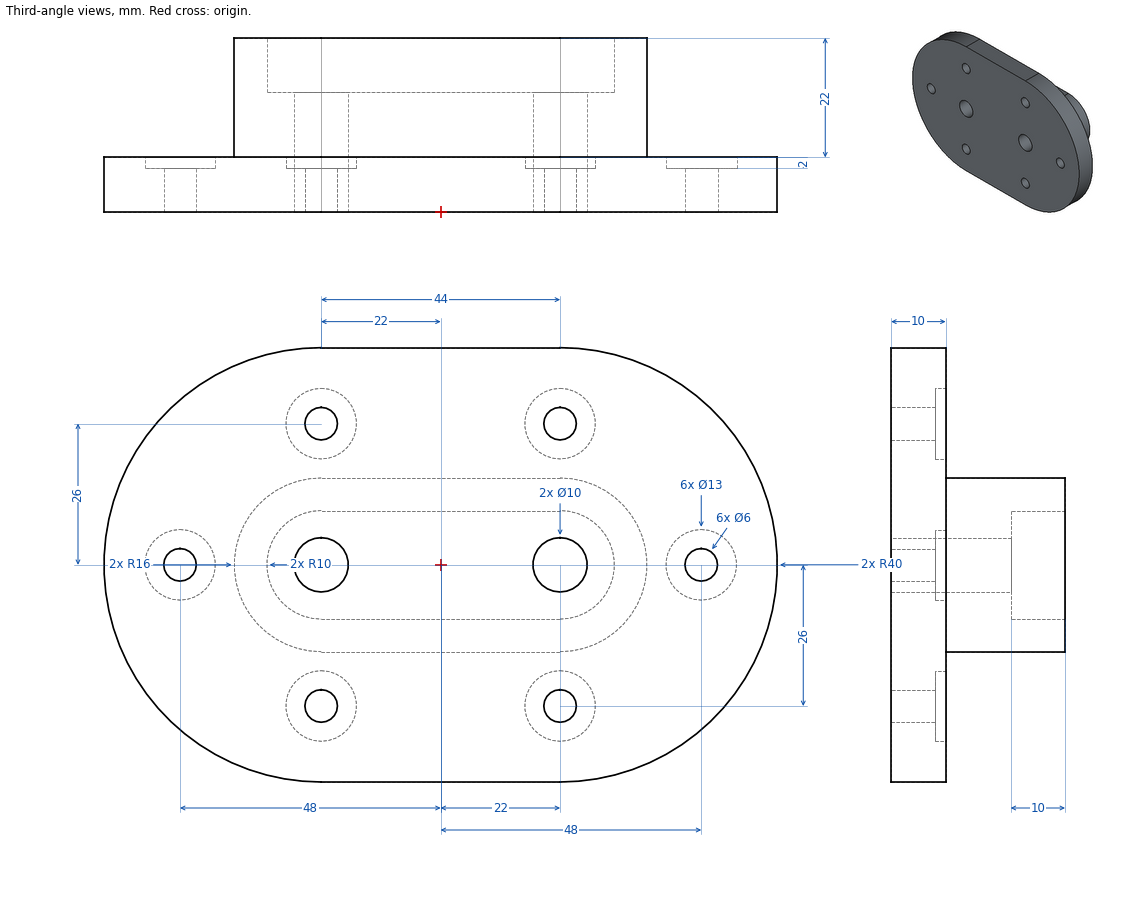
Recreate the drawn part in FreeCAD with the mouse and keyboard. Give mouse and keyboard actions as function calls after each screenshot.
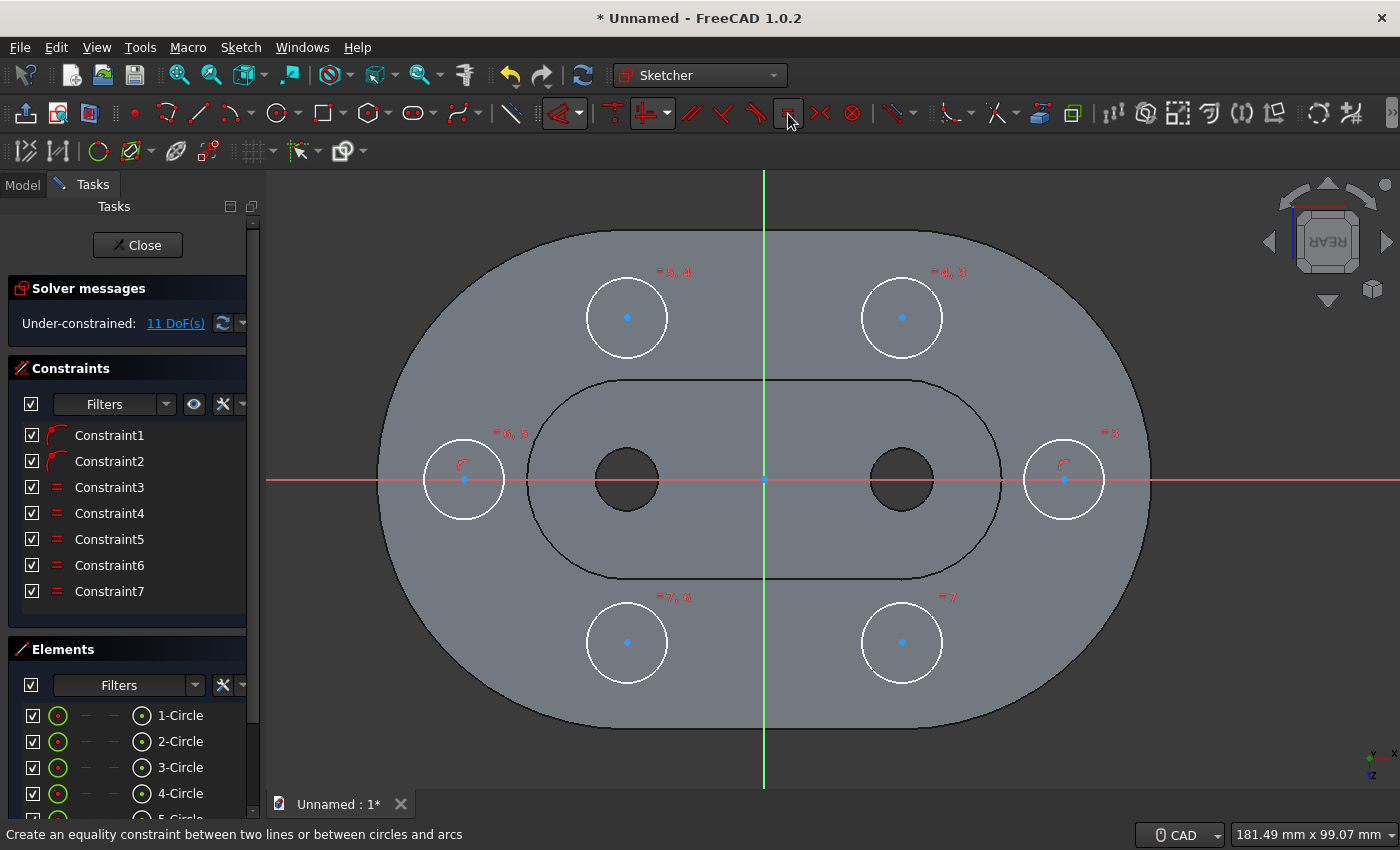
click(902, 318)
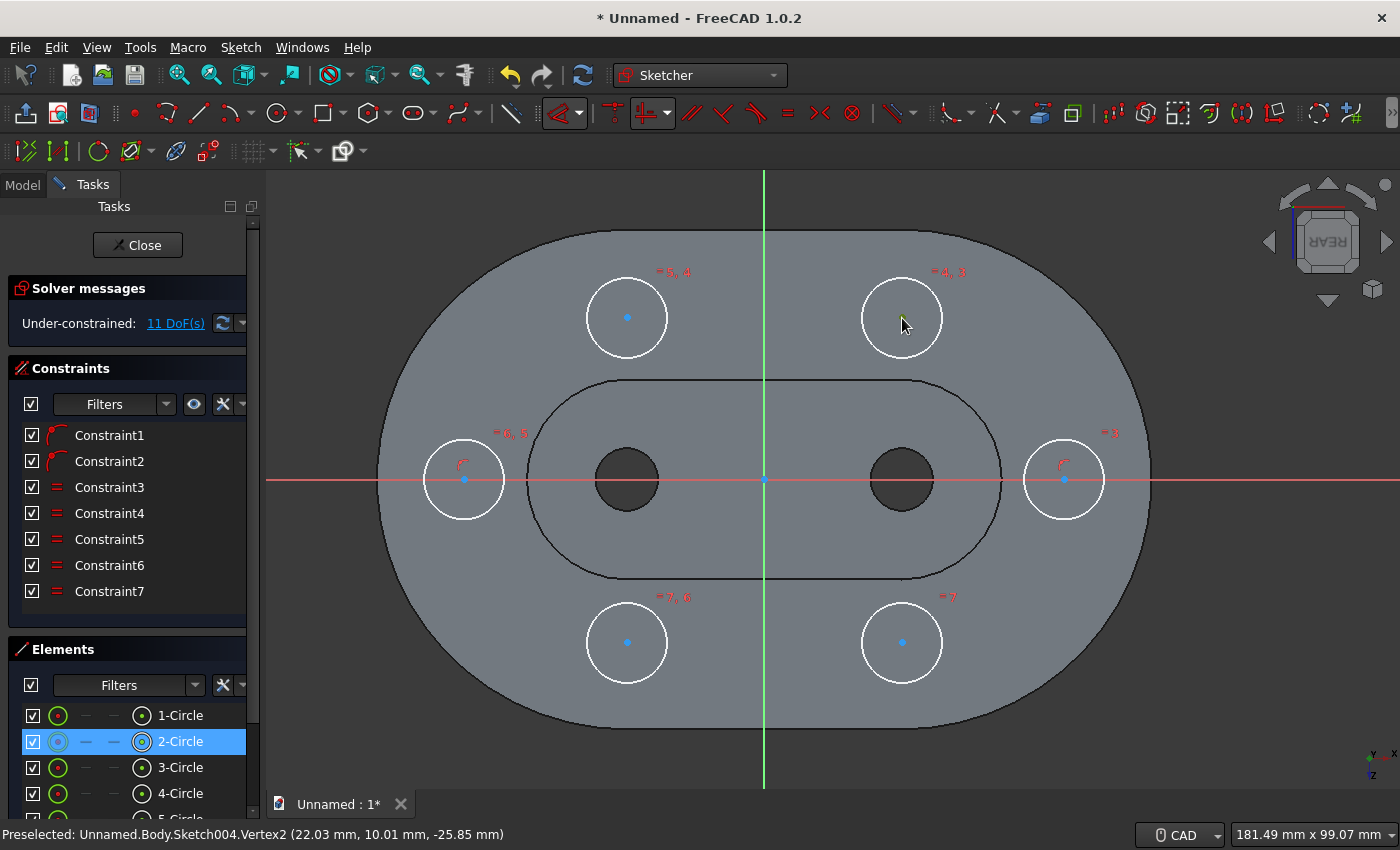
click(627, 318)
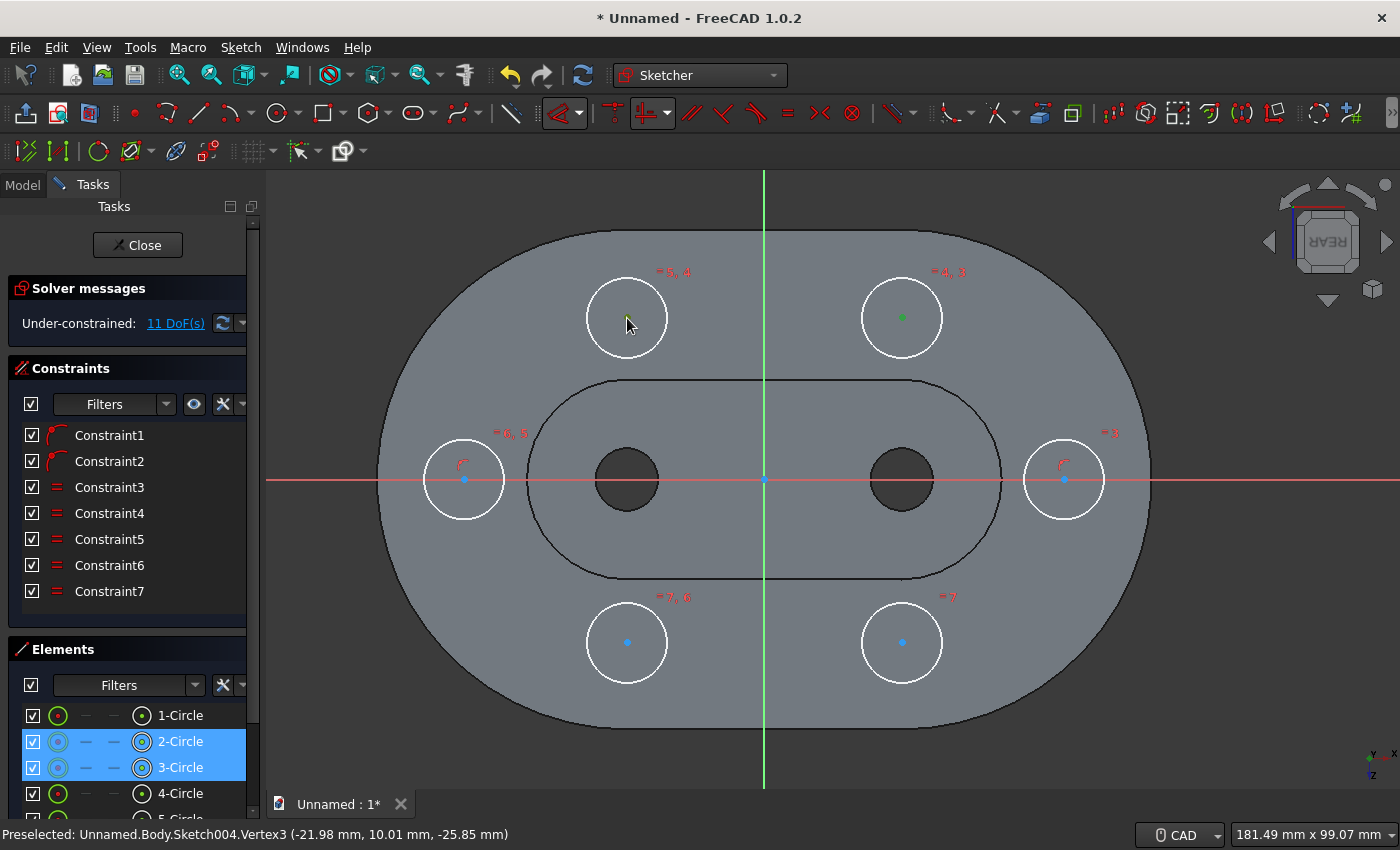
key(h)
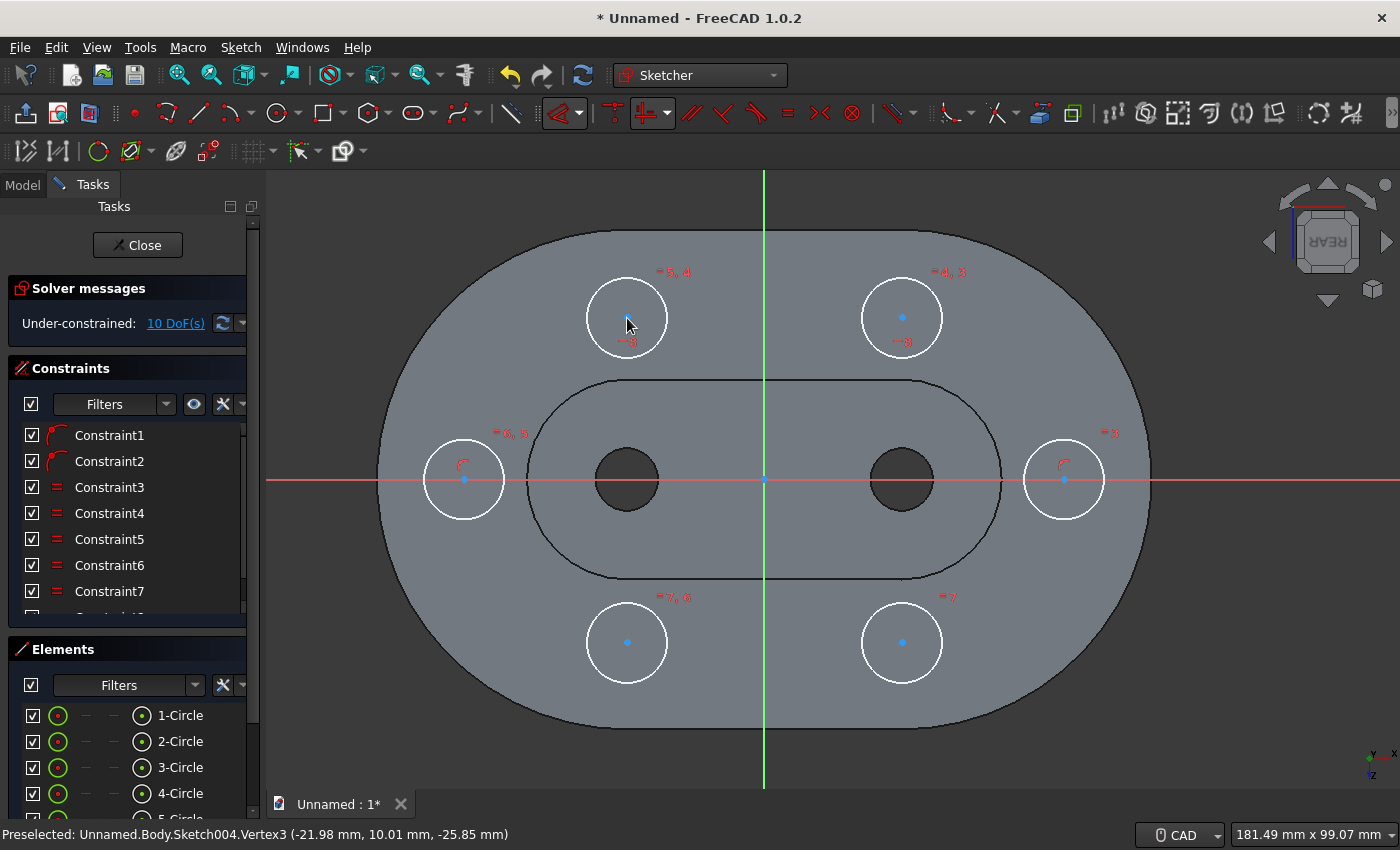
click(627, 318)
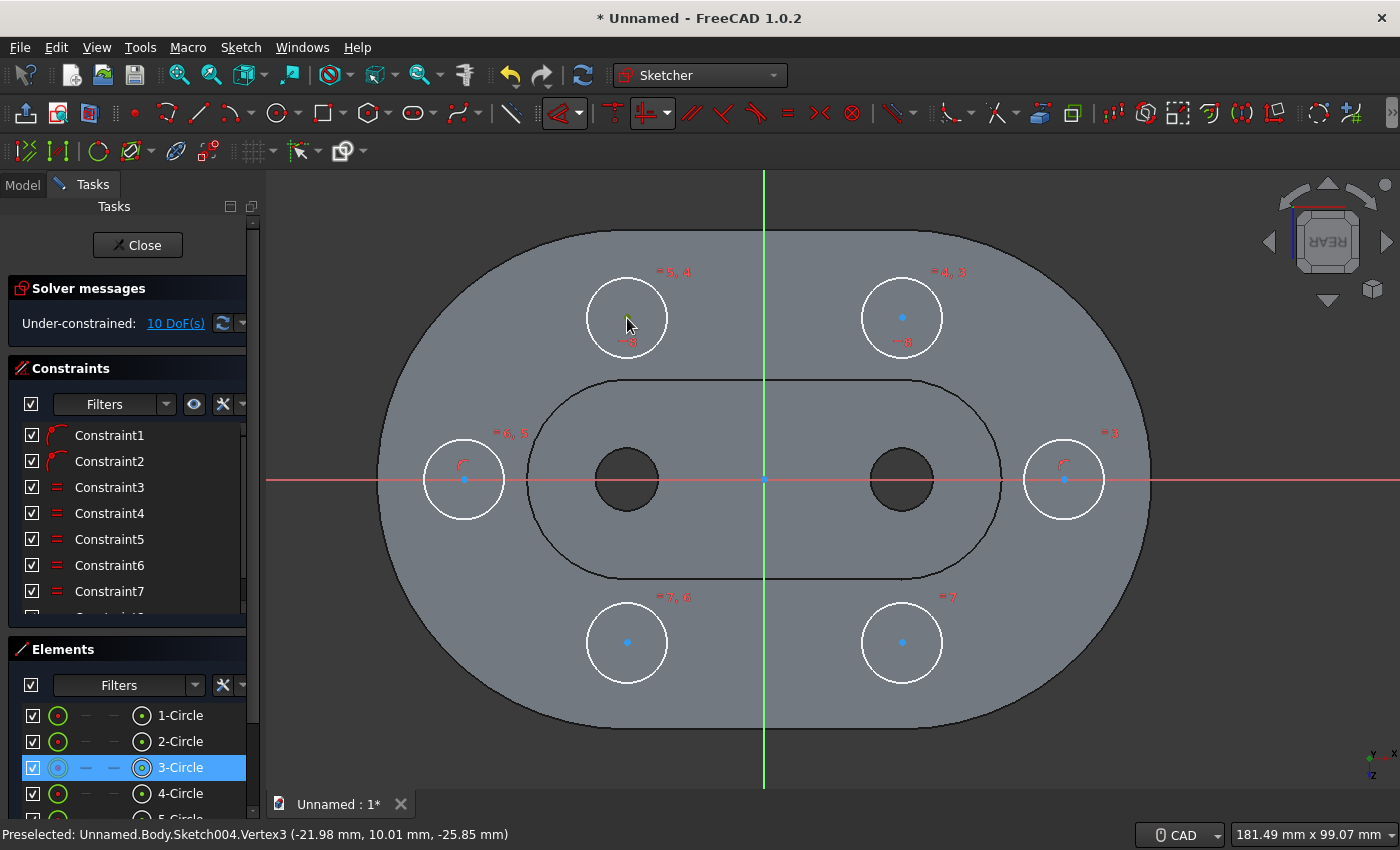
click(627, 643)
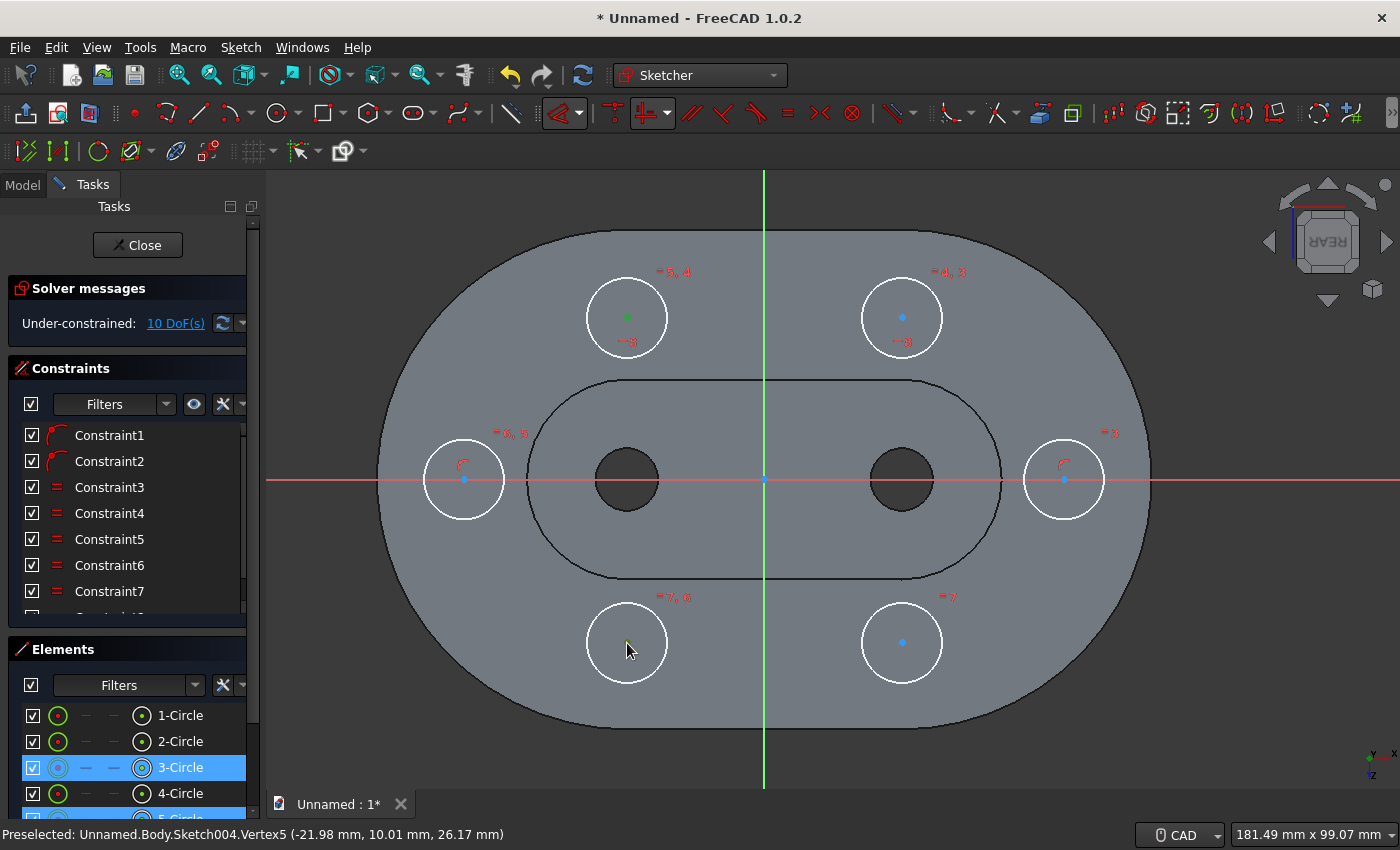
key(v)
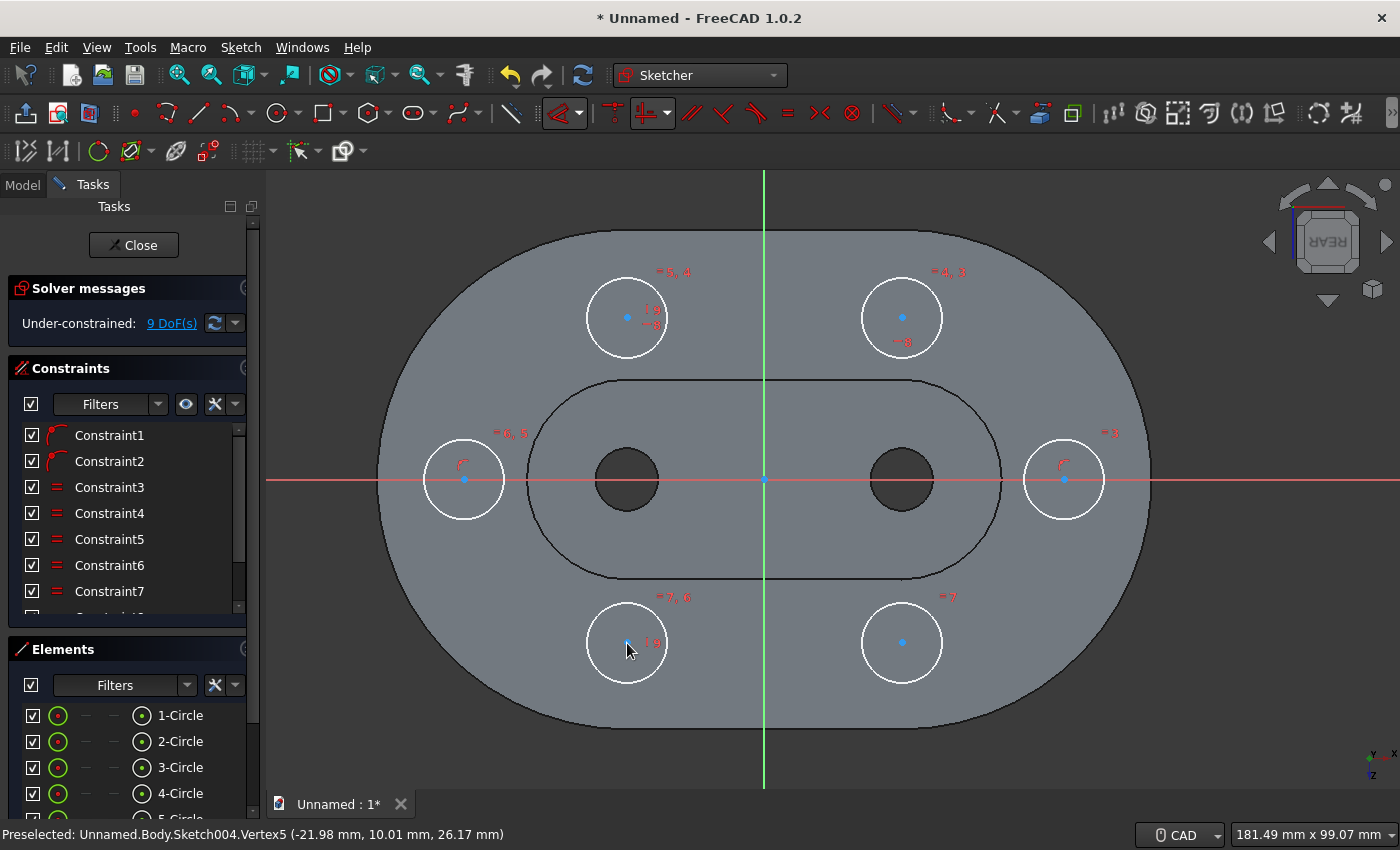
click(902, 318)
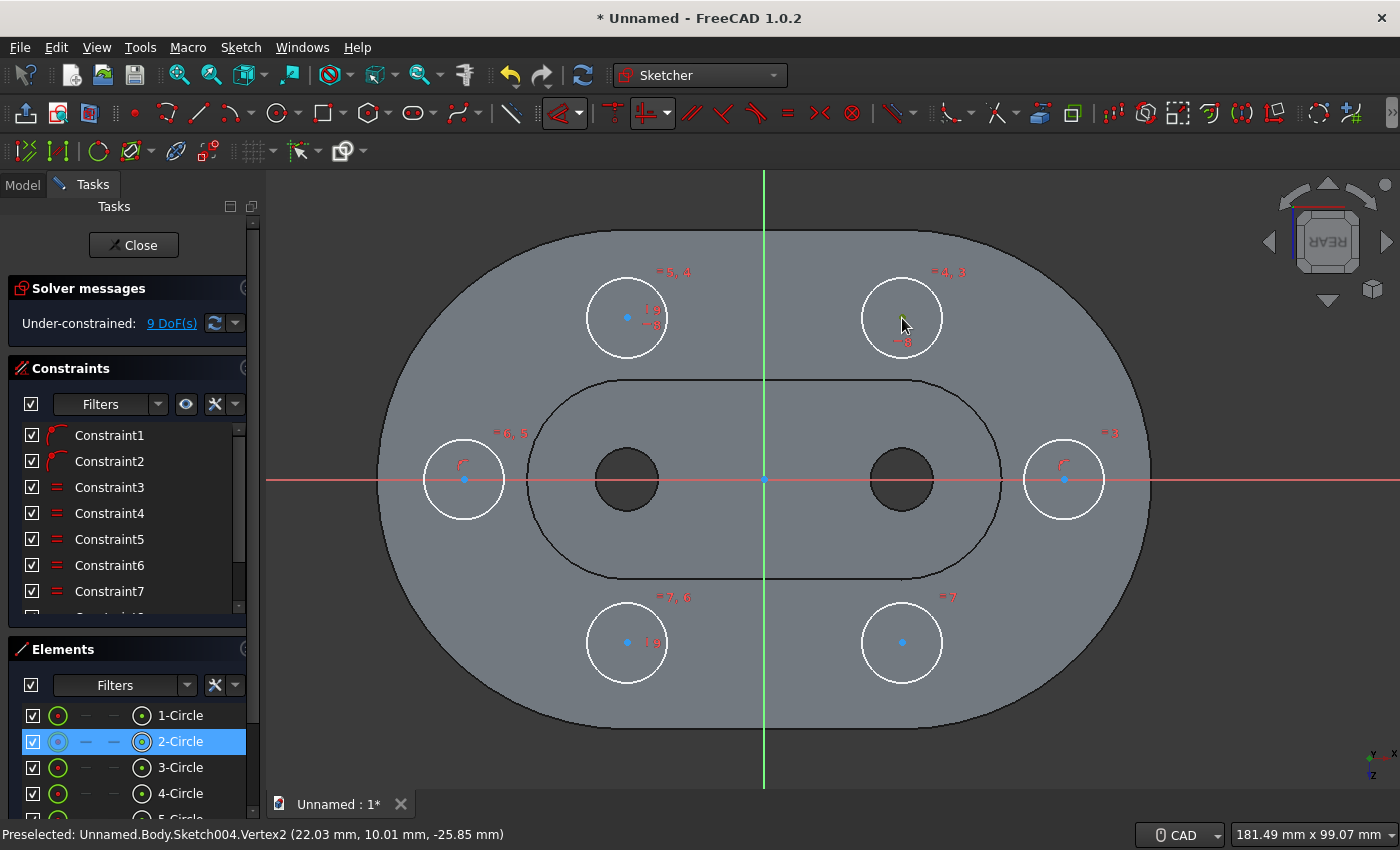
click(902, 643)